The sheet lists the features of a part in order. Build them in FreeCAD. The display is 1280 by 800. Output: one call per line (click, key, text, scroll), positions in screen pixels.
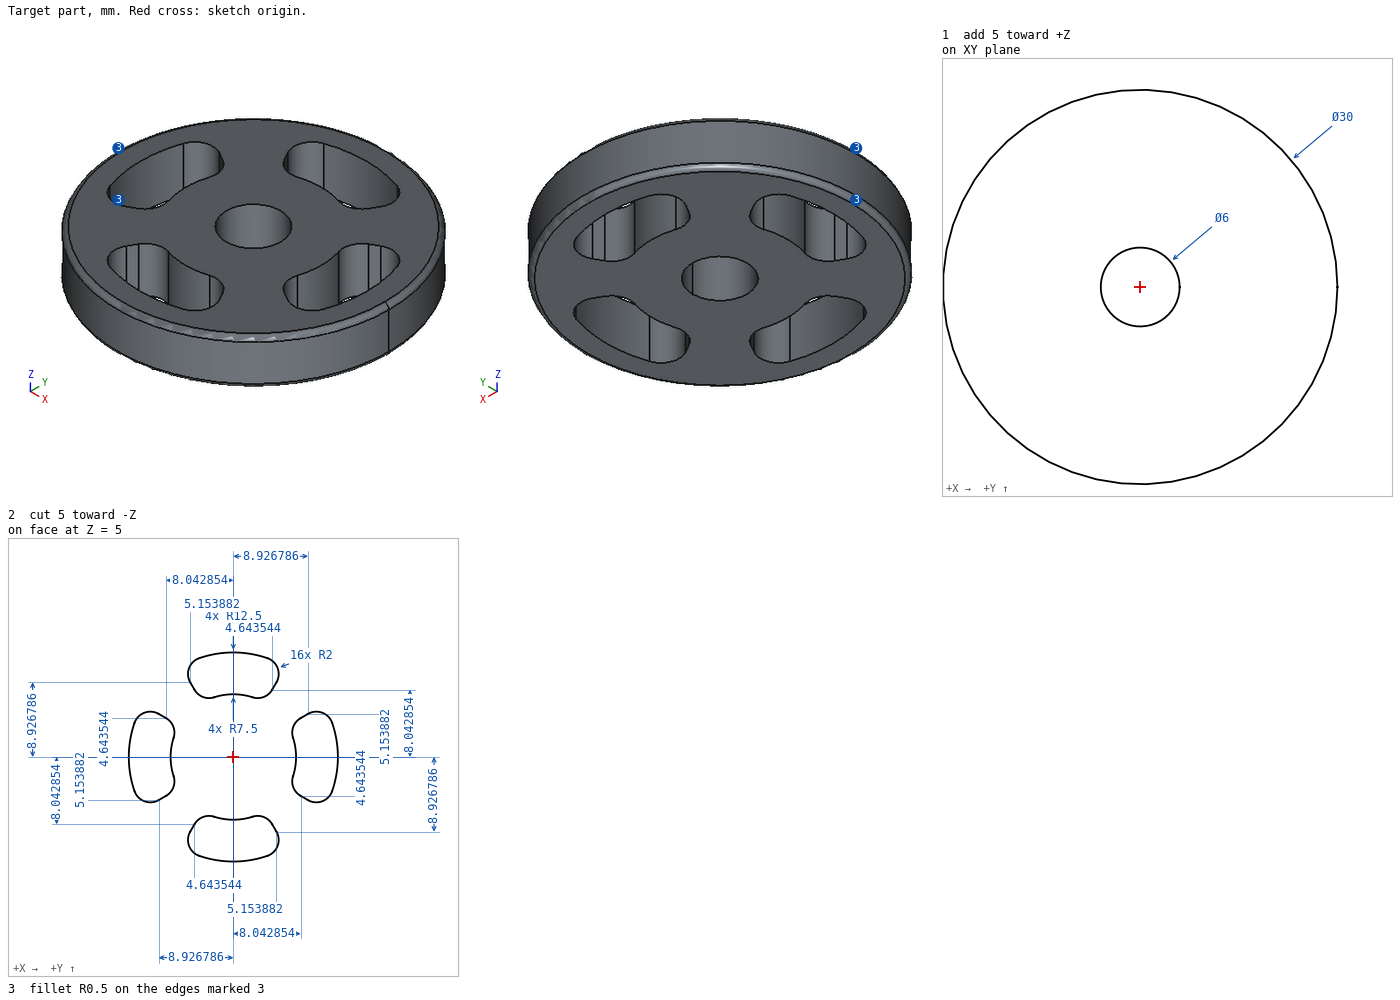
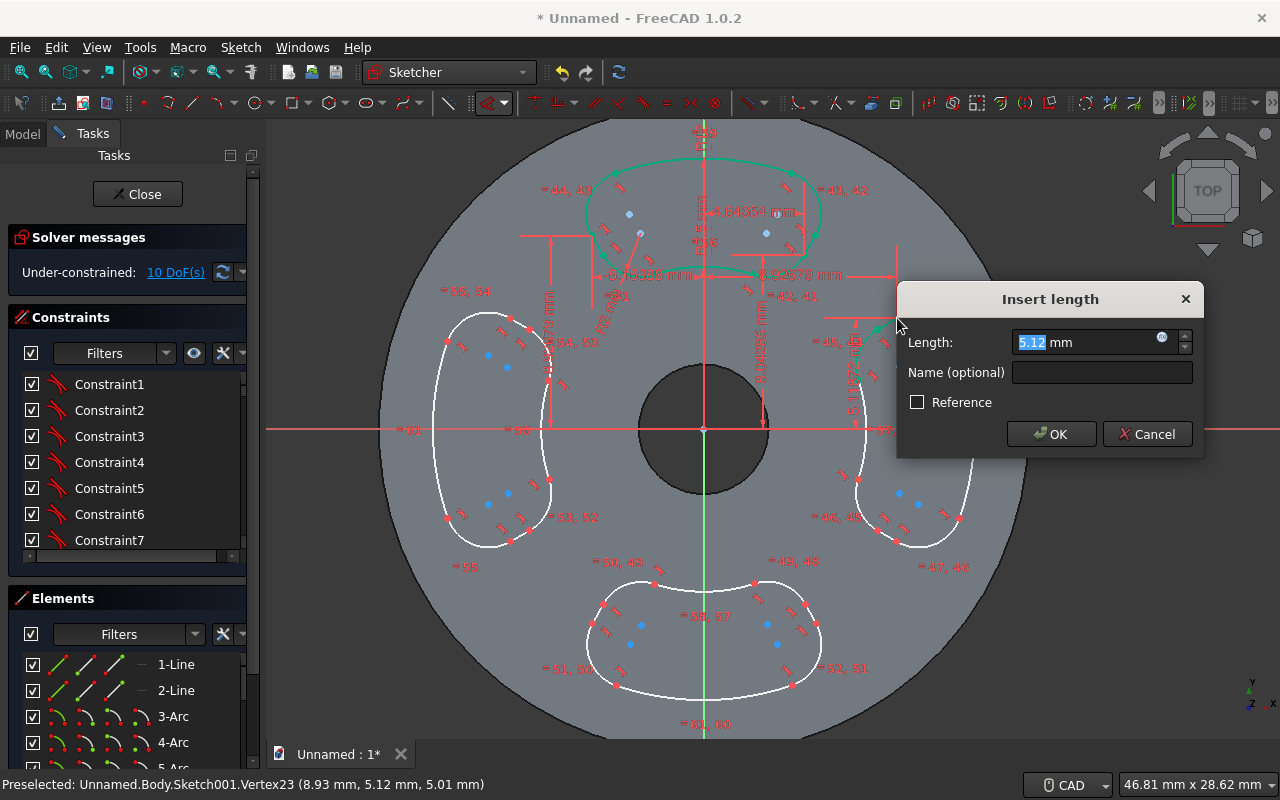
text(5.153882)
key(Return)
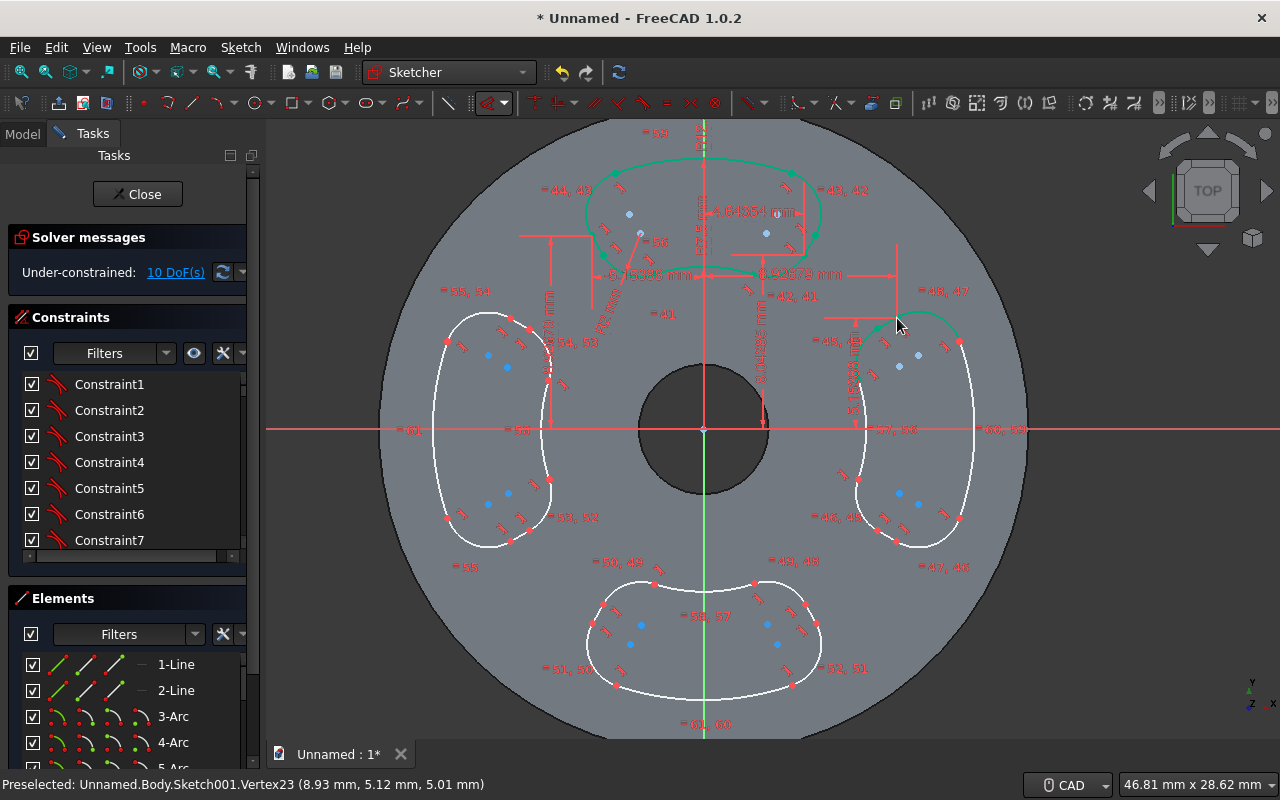
click(878, 531)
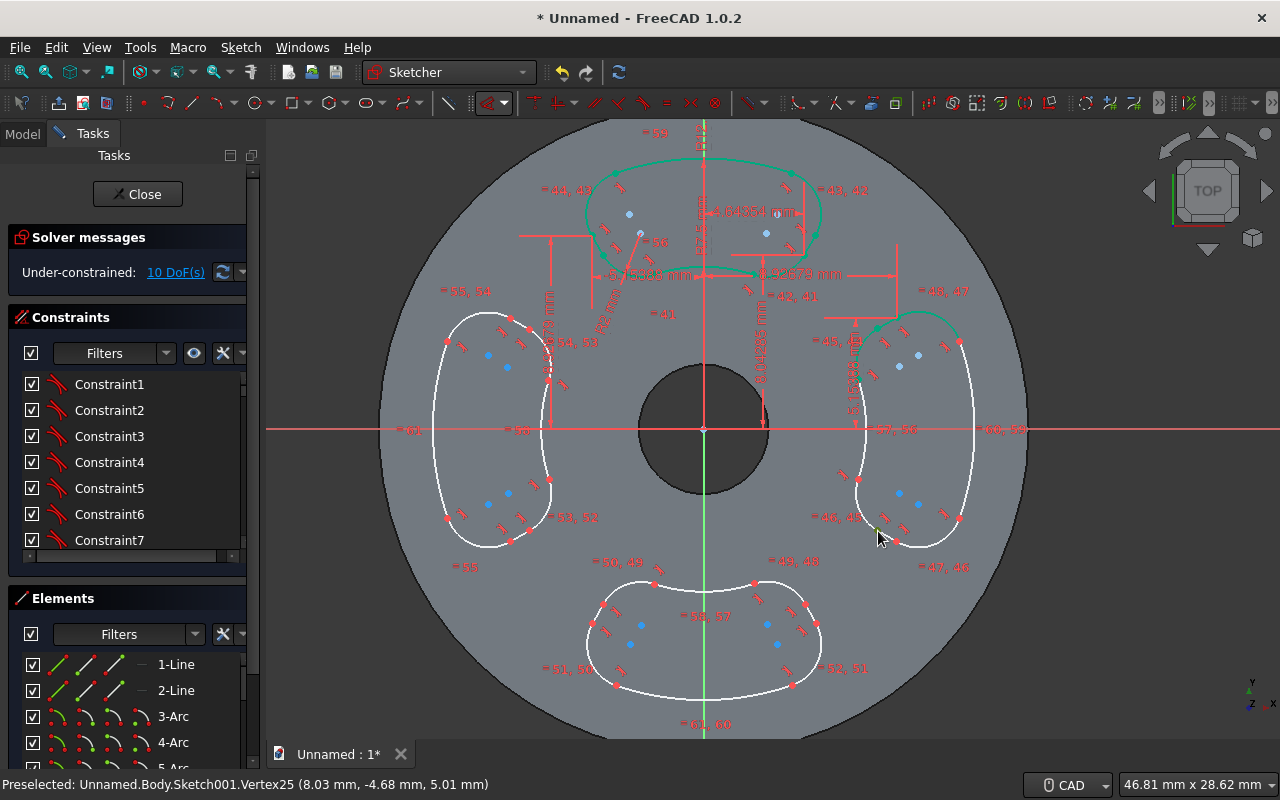
key(l)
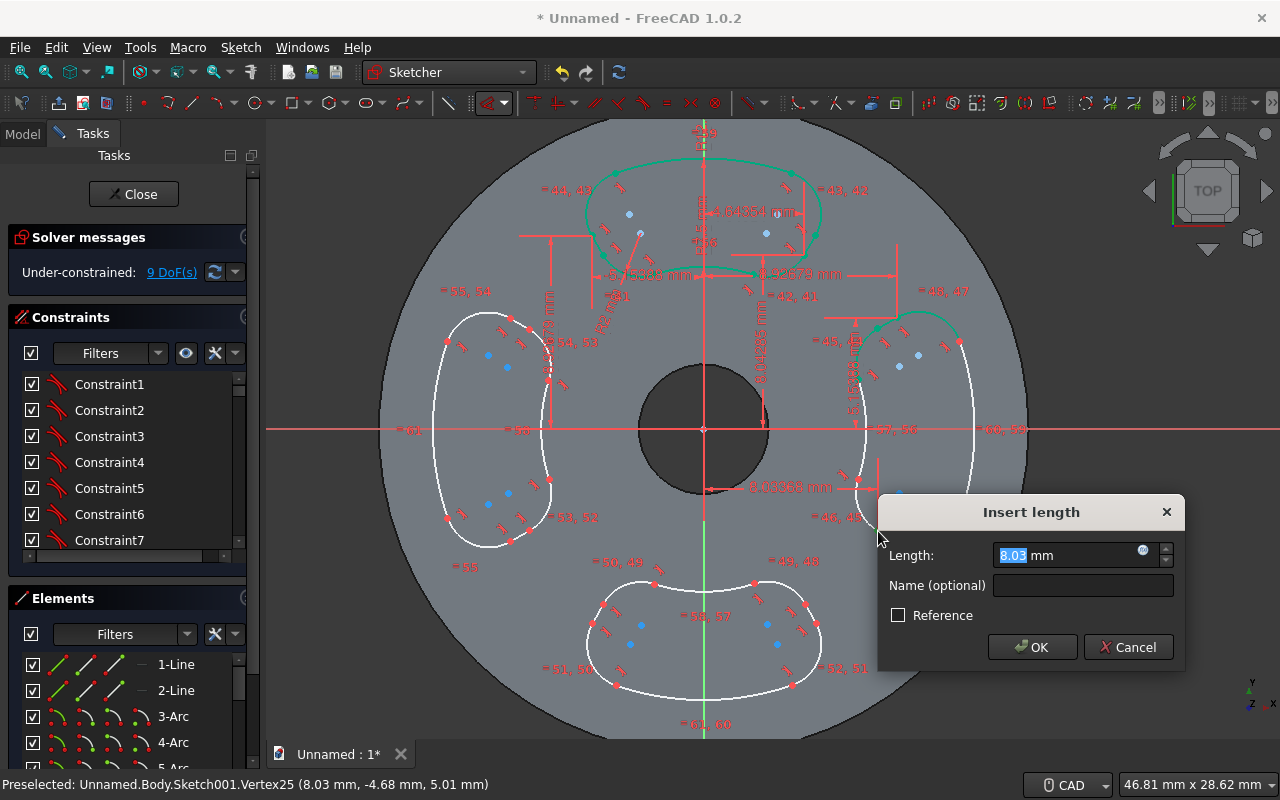
text(8.042854)
key(Return)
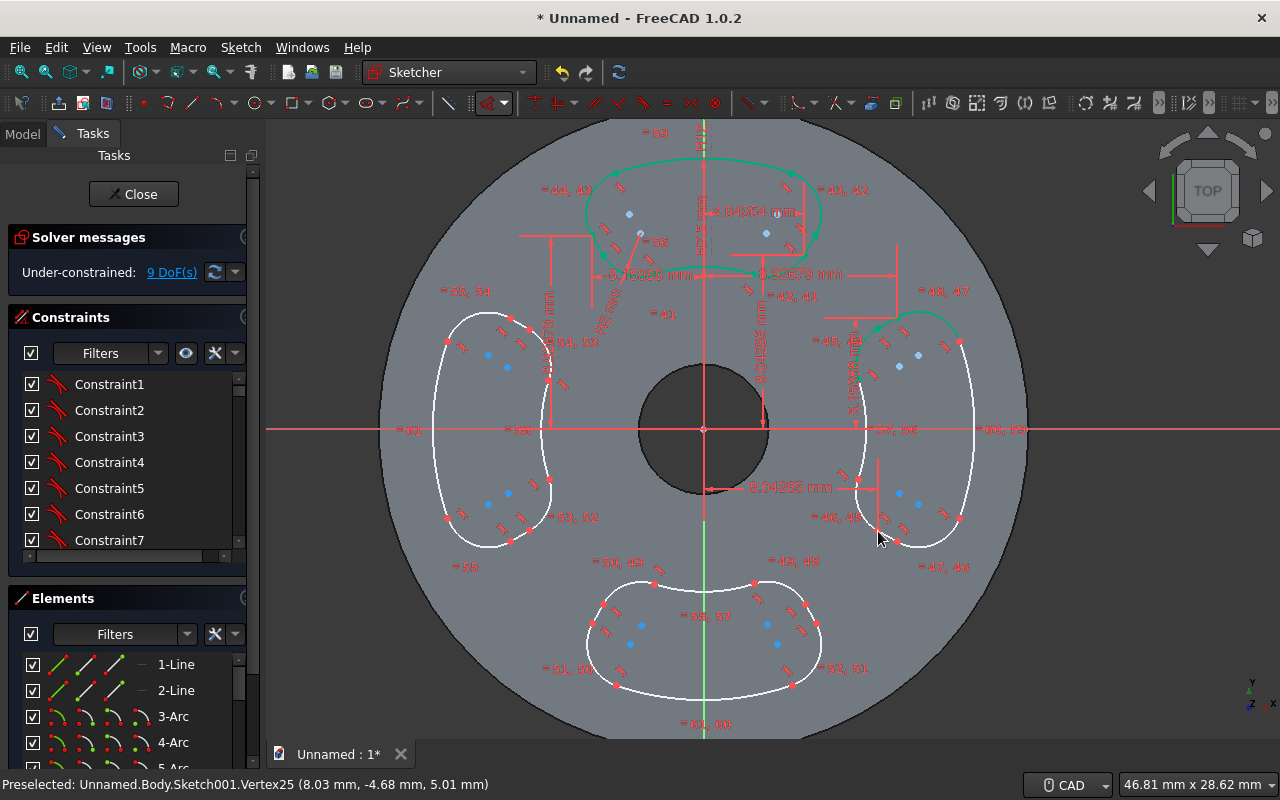
click(878, 531)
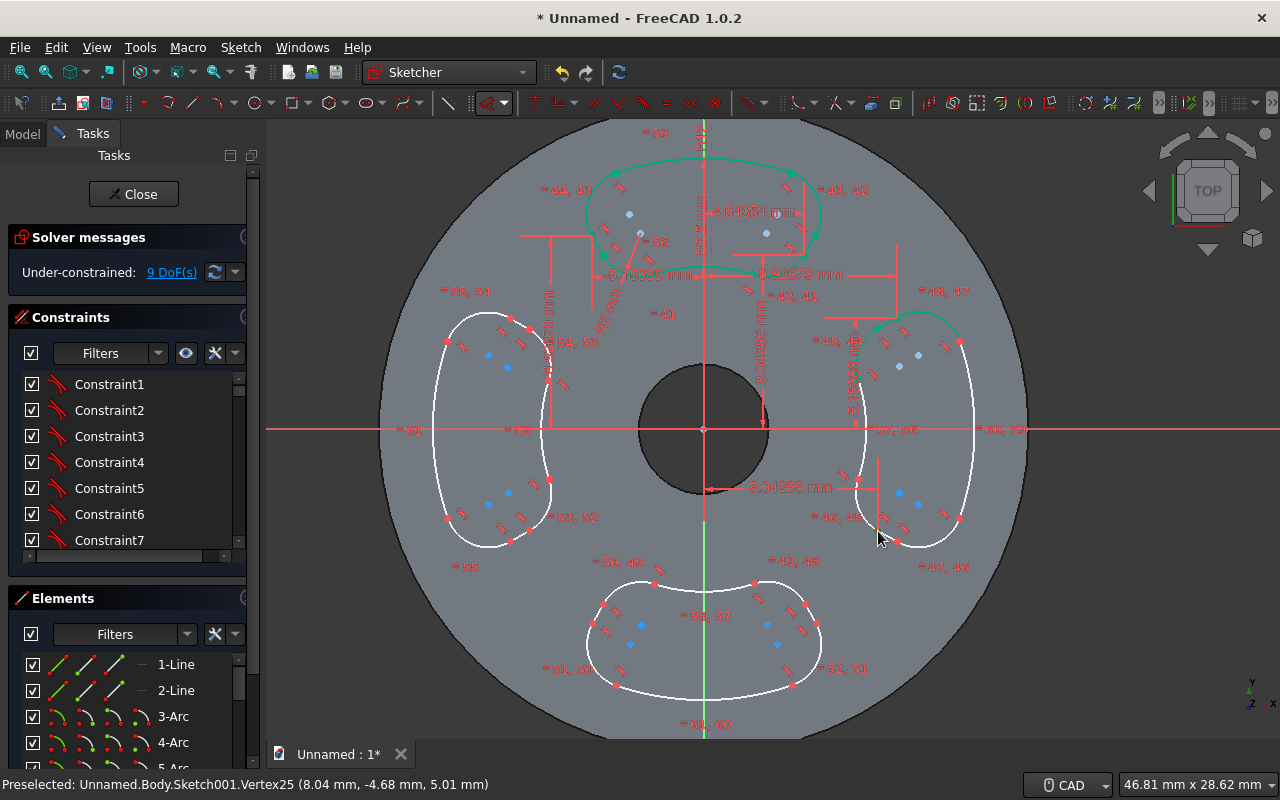
click(506, 104)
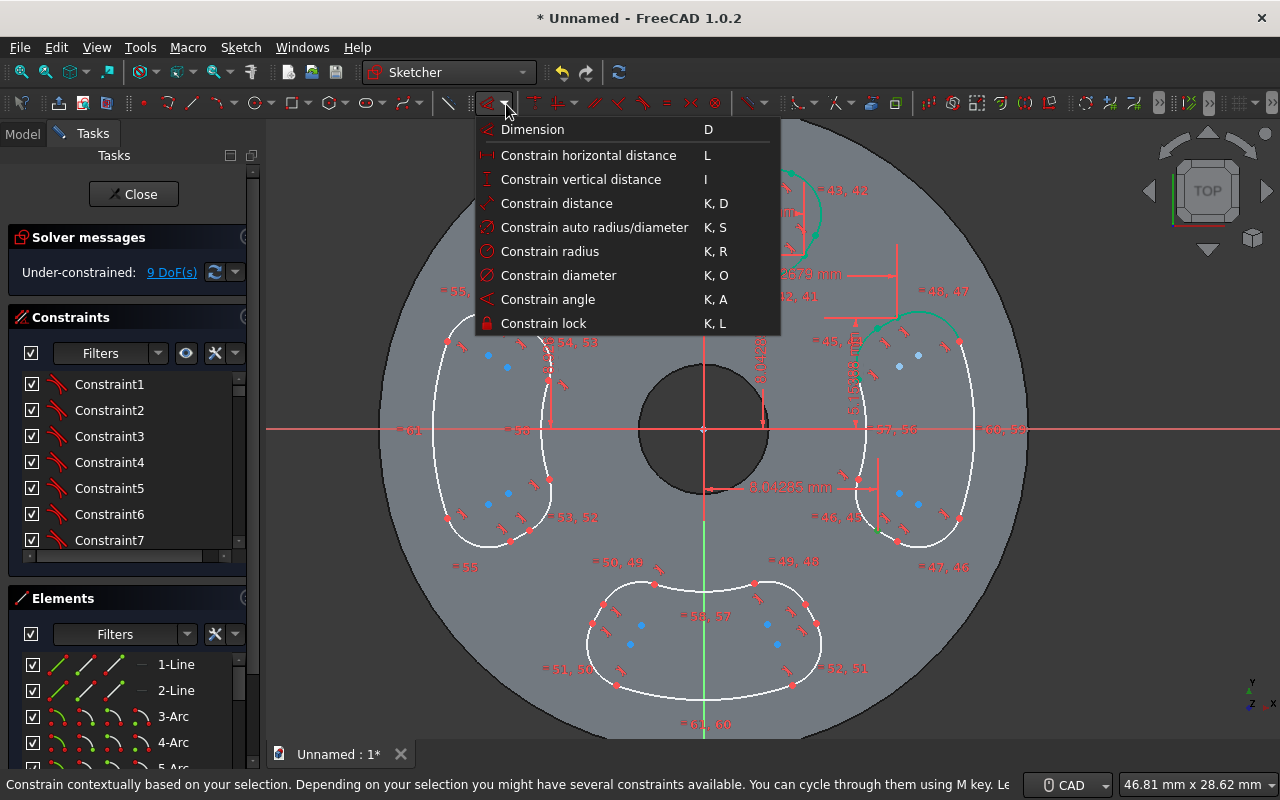
click(628, 179)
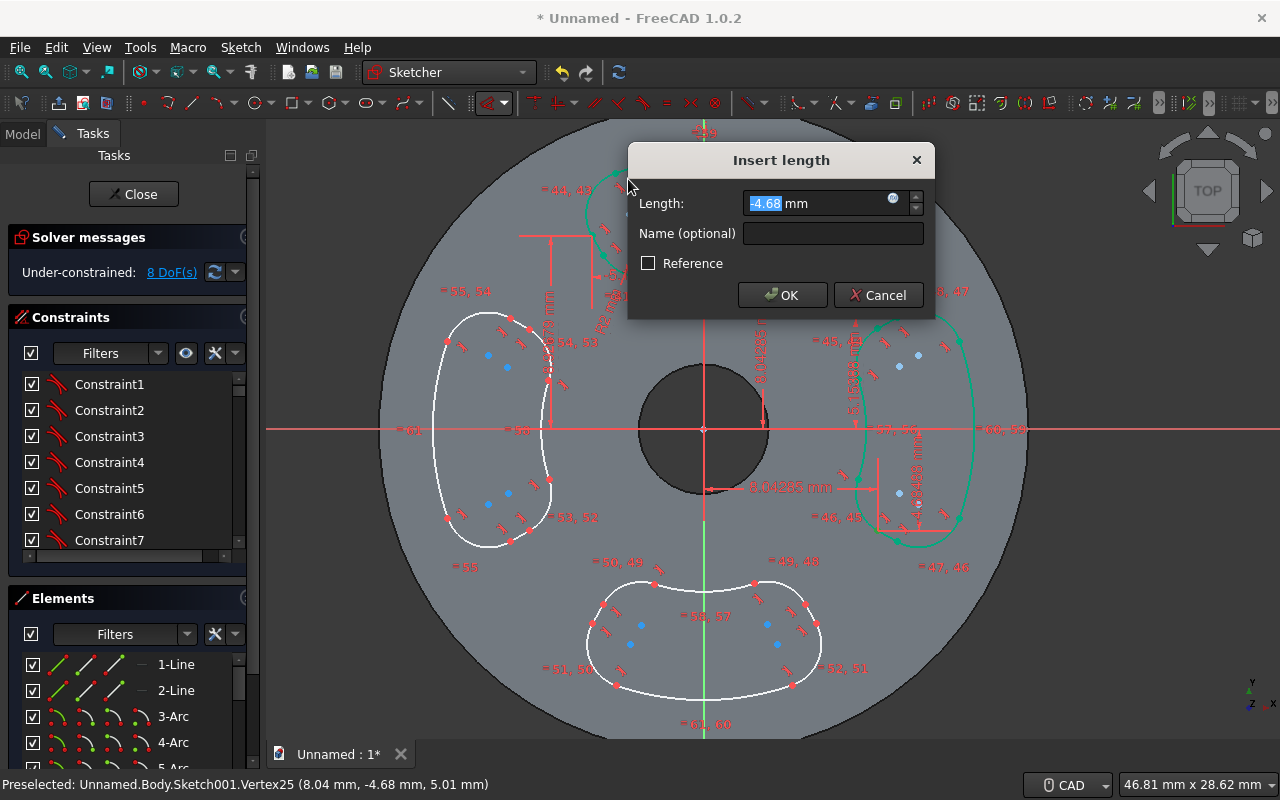
text(-4.643544)
key(Return)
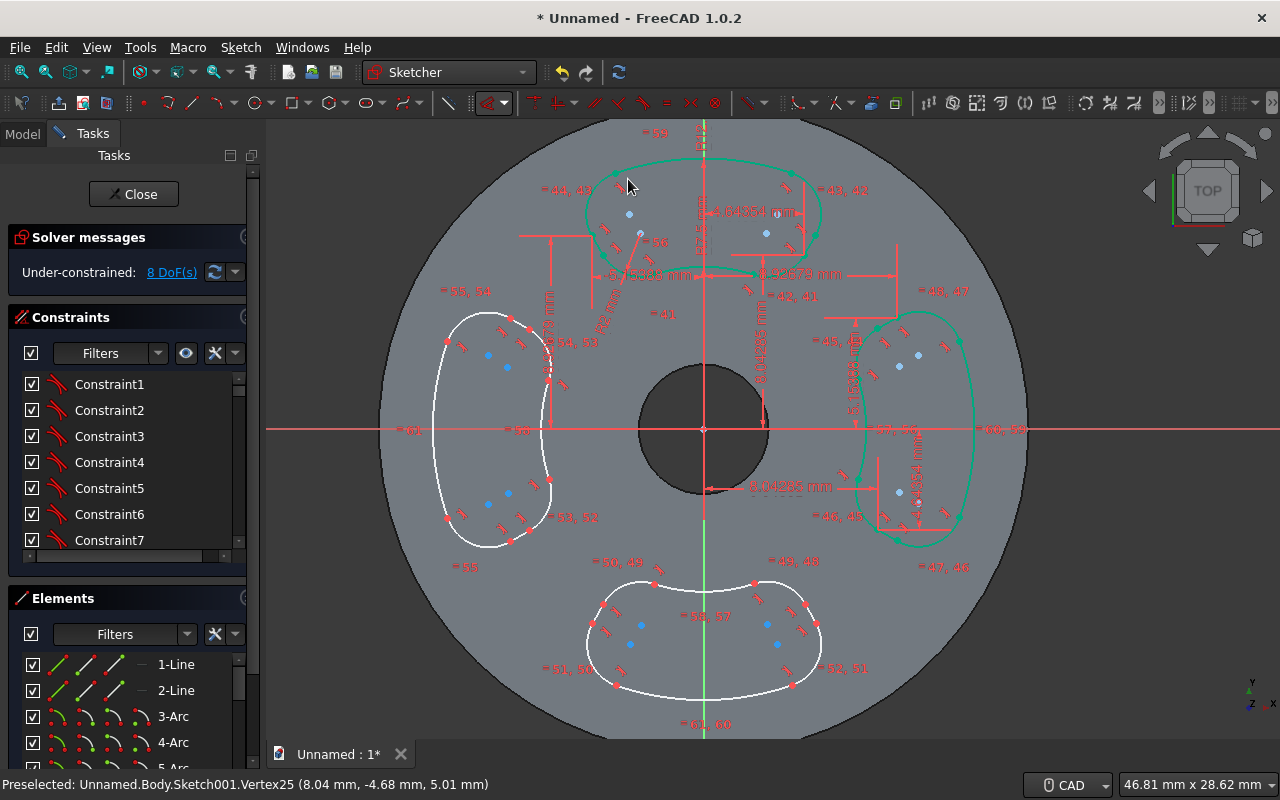
click(816, 623)